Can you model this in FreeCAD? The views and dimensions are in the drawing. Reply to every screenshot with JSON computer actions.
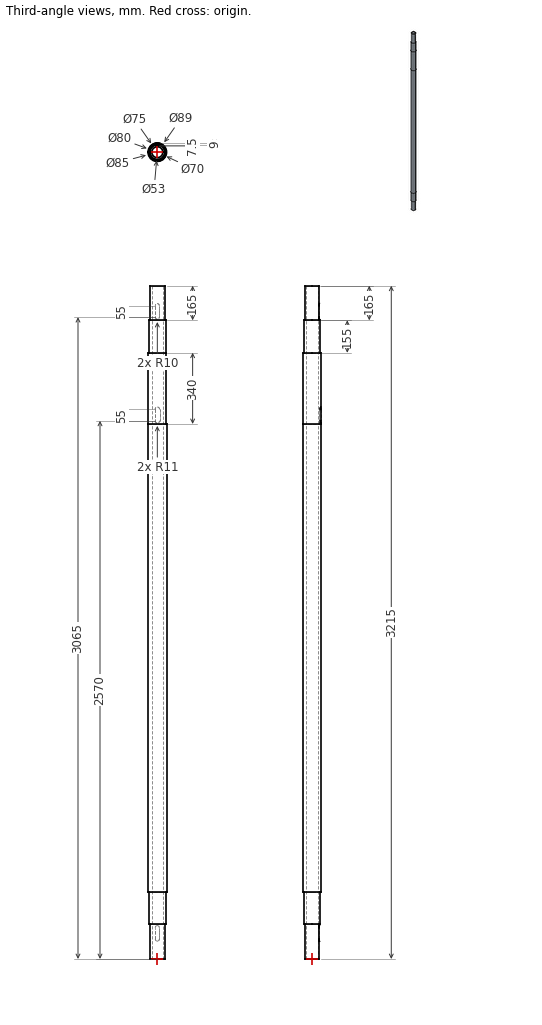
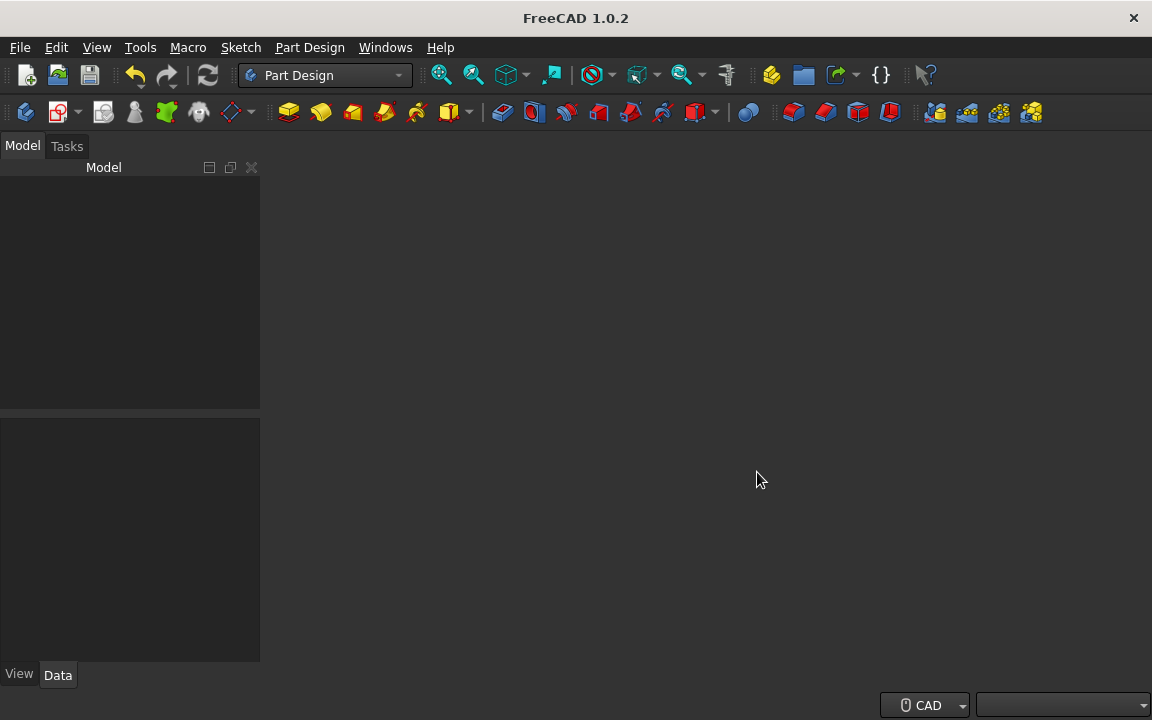
{"action": "left_click", "coordinate": [26, 76]}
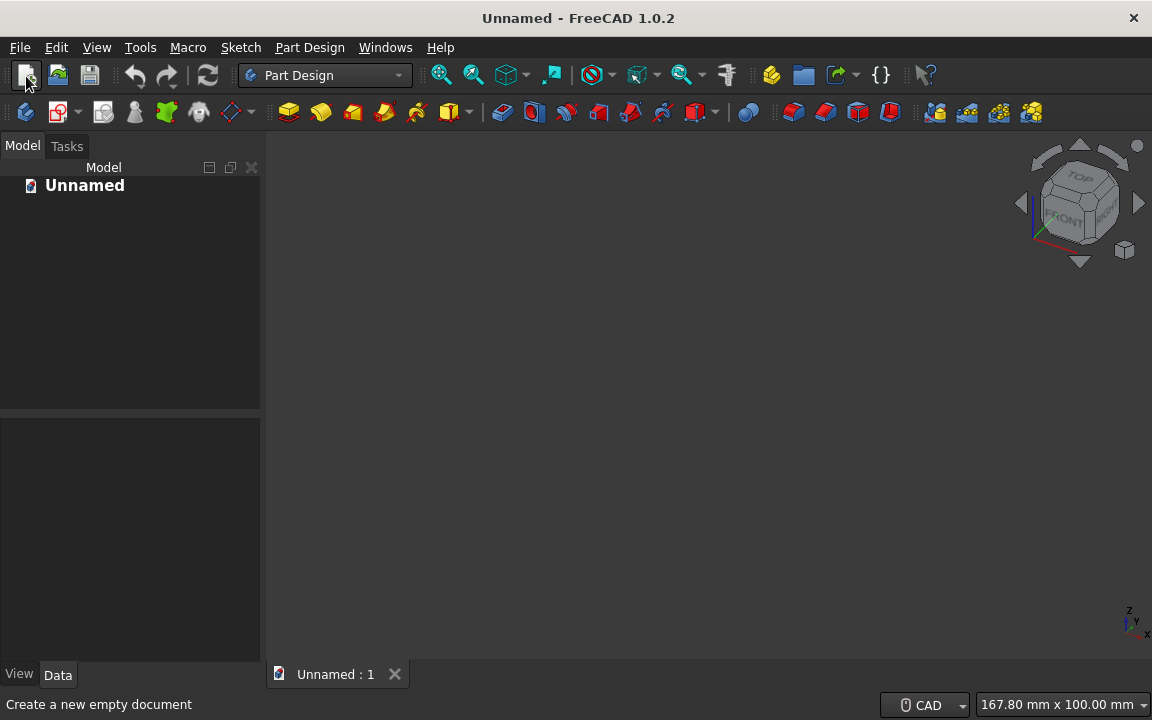
{"action": "left_click", "coordinate": [58, 112]}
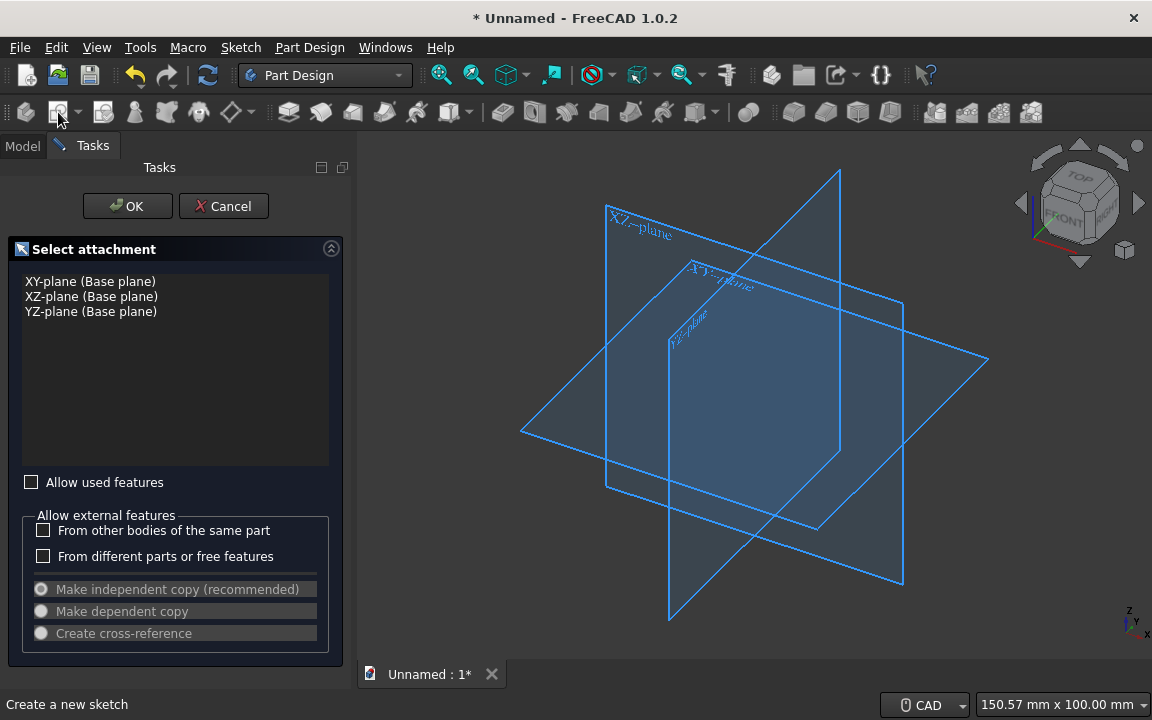
{"action": "left_click", "coordinate": [82, 282]}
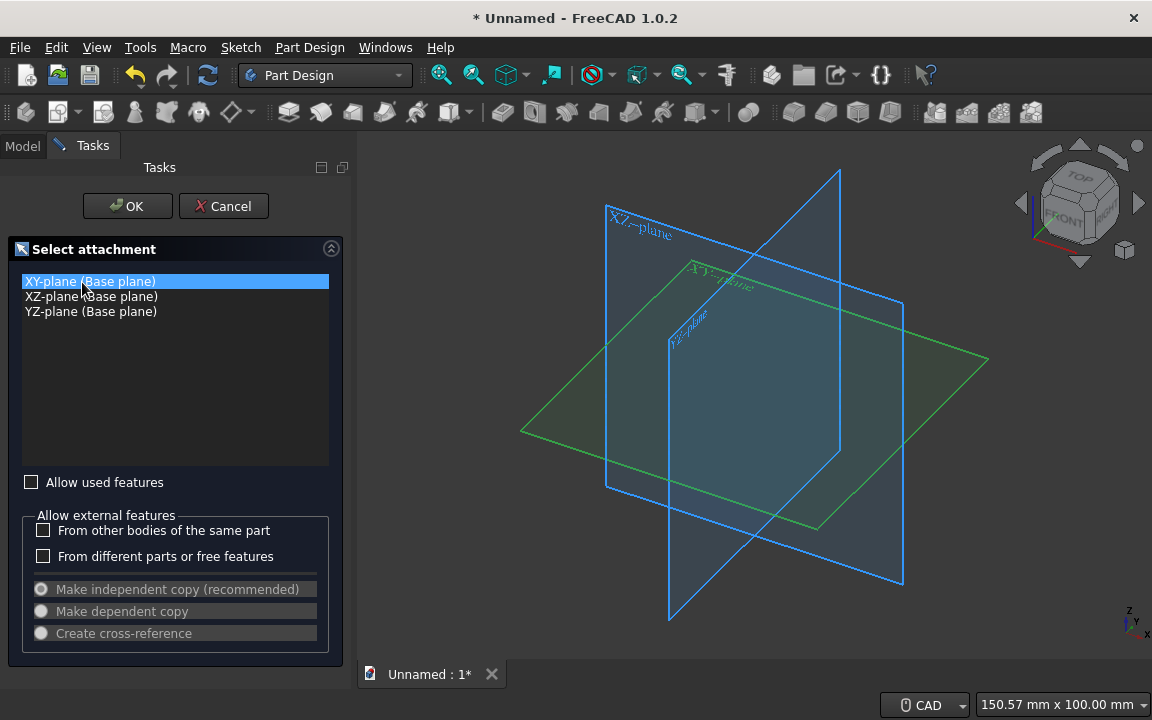
{"action": "left_click", "coordinate": [128, 206]}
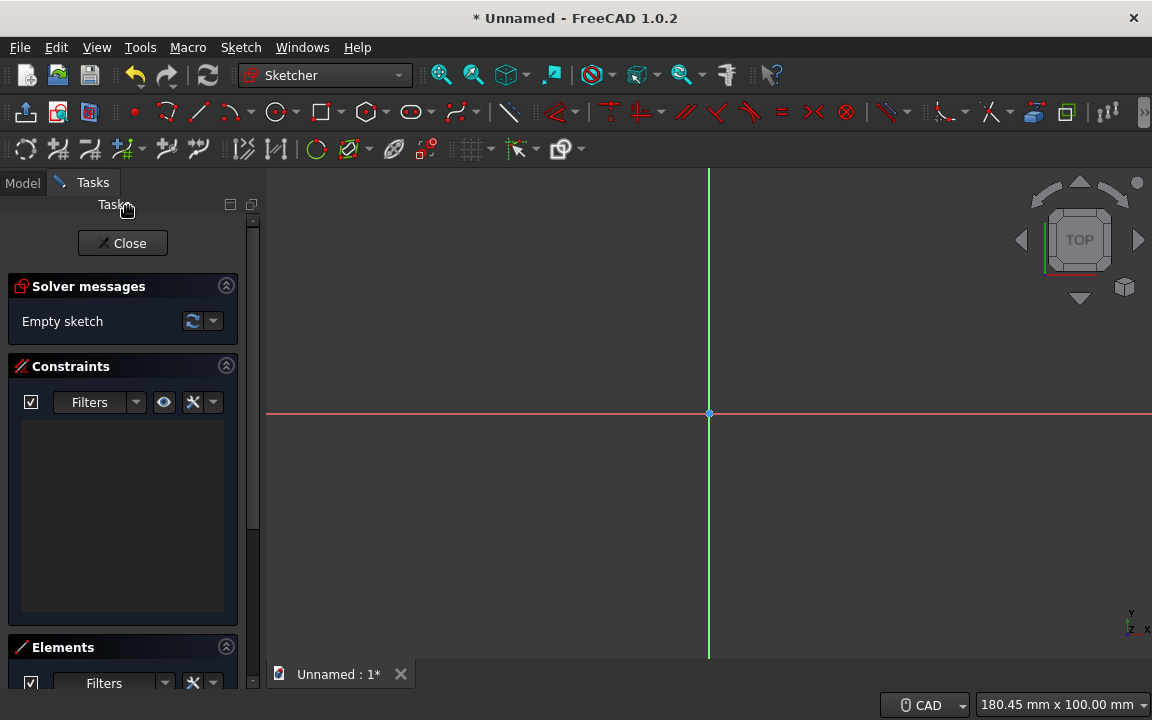
{"action": "scroll", "coordinate": [501, 414], "scroll_direction": "down", "scroll_amount": 2}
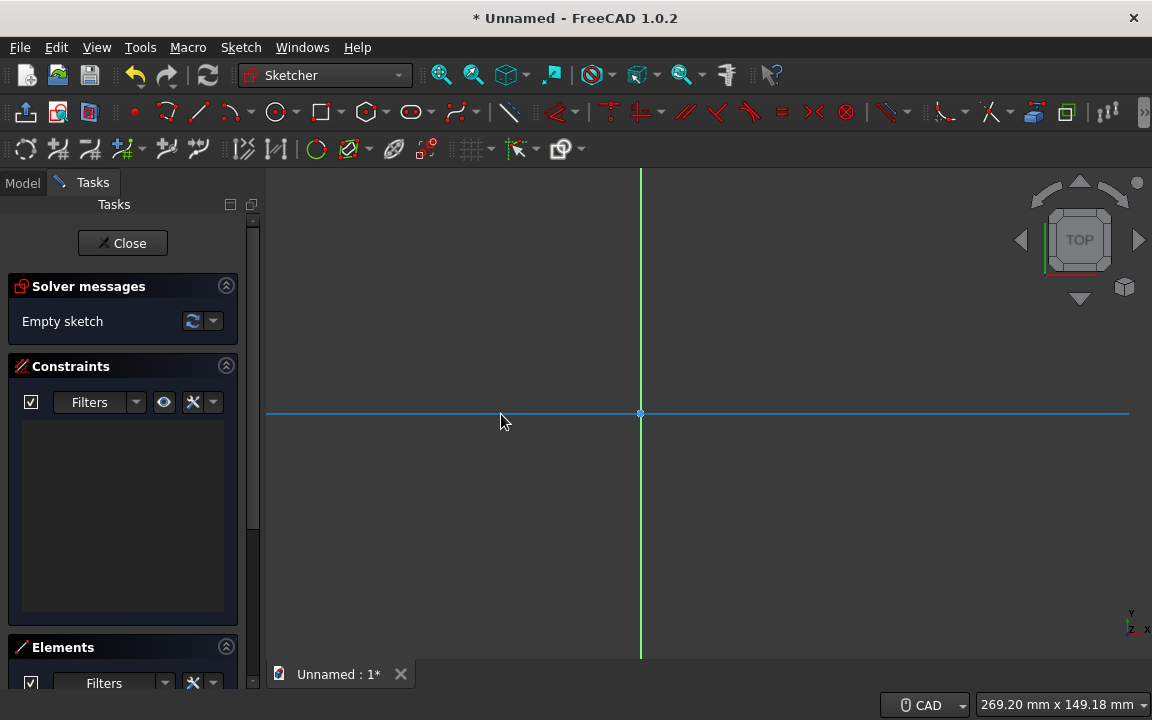
{"action": "left_click", "coordinate": [276, 112]}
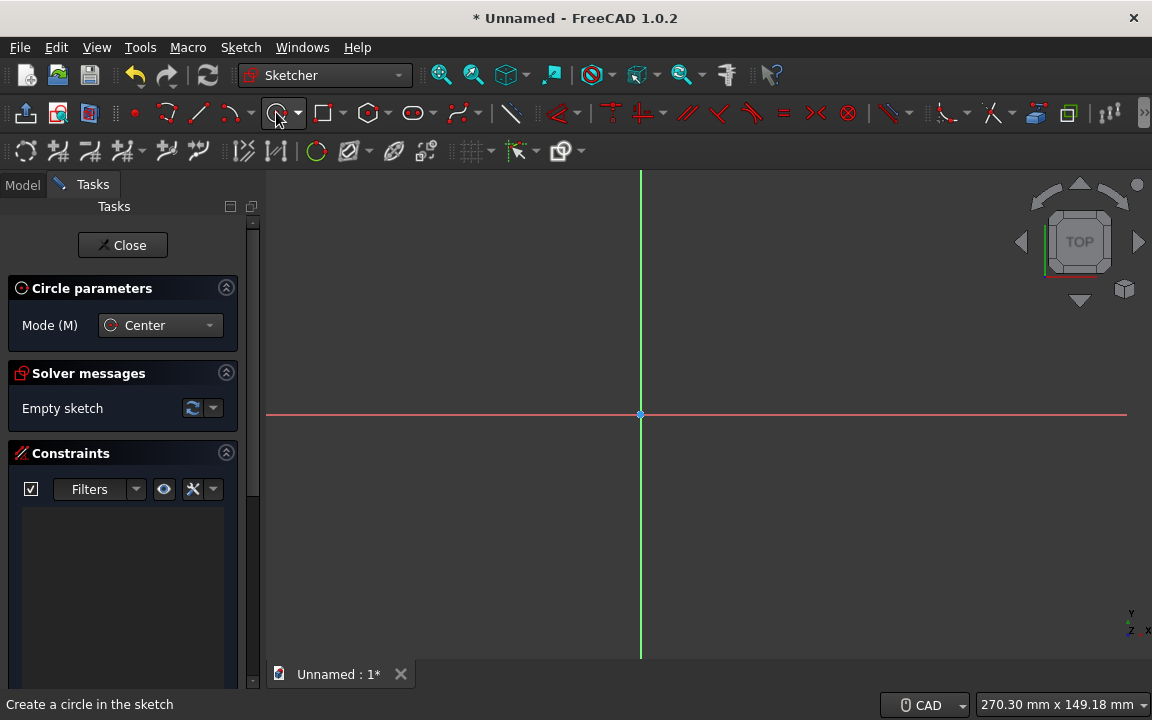
{"action": "left_click", "coordinate": [641, 415]}
{"action": "mouse_move", "coordinate": [744, 312]}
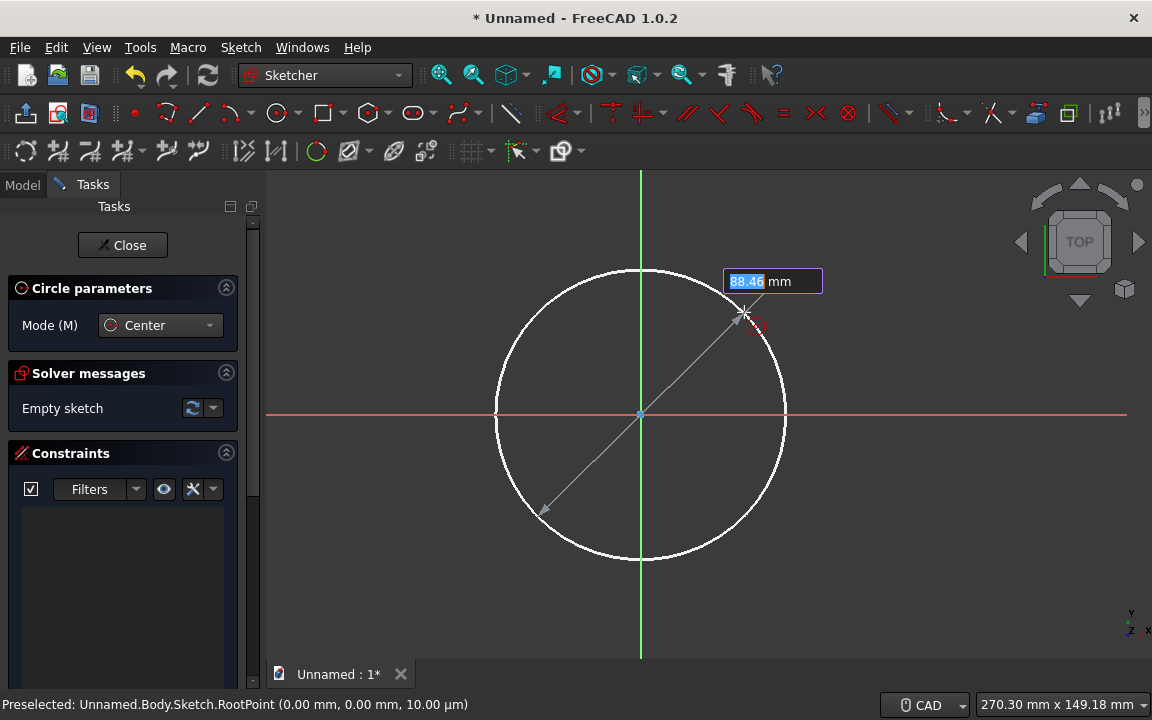
{"action": "type", "text": "89"}
{"action": "key", "text": "Return"}
{"action": "key", "text": "Escape"}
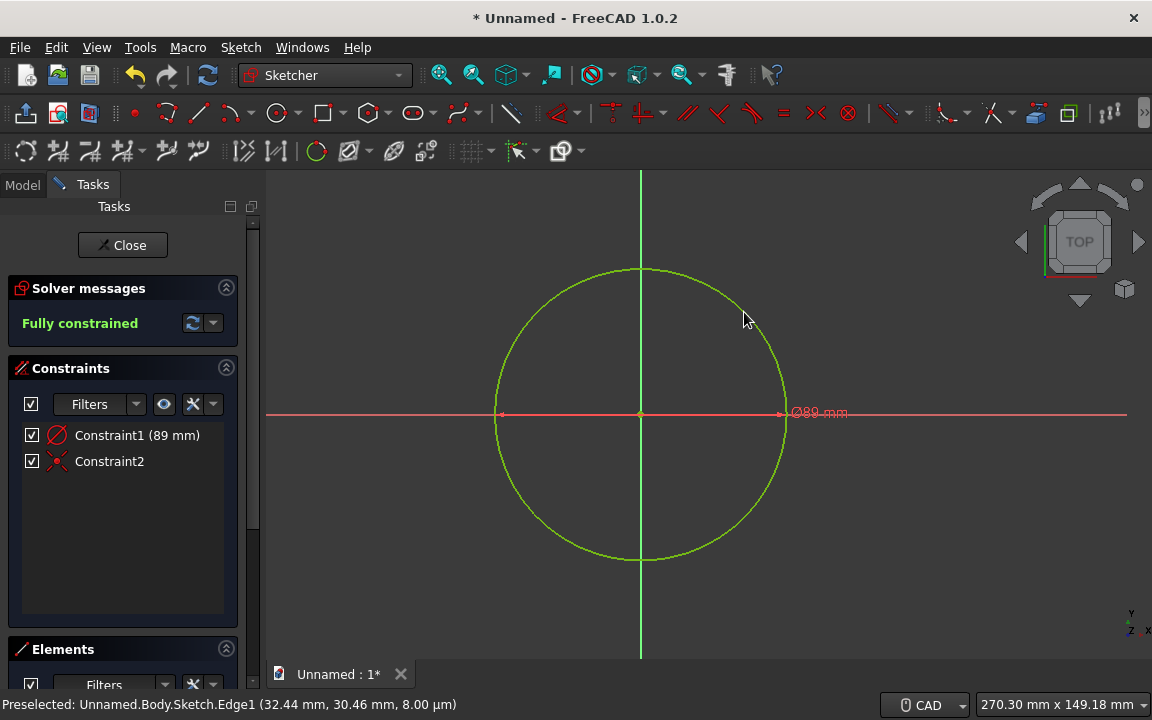
{"action": "left_click", "coordinate": [123, 245]}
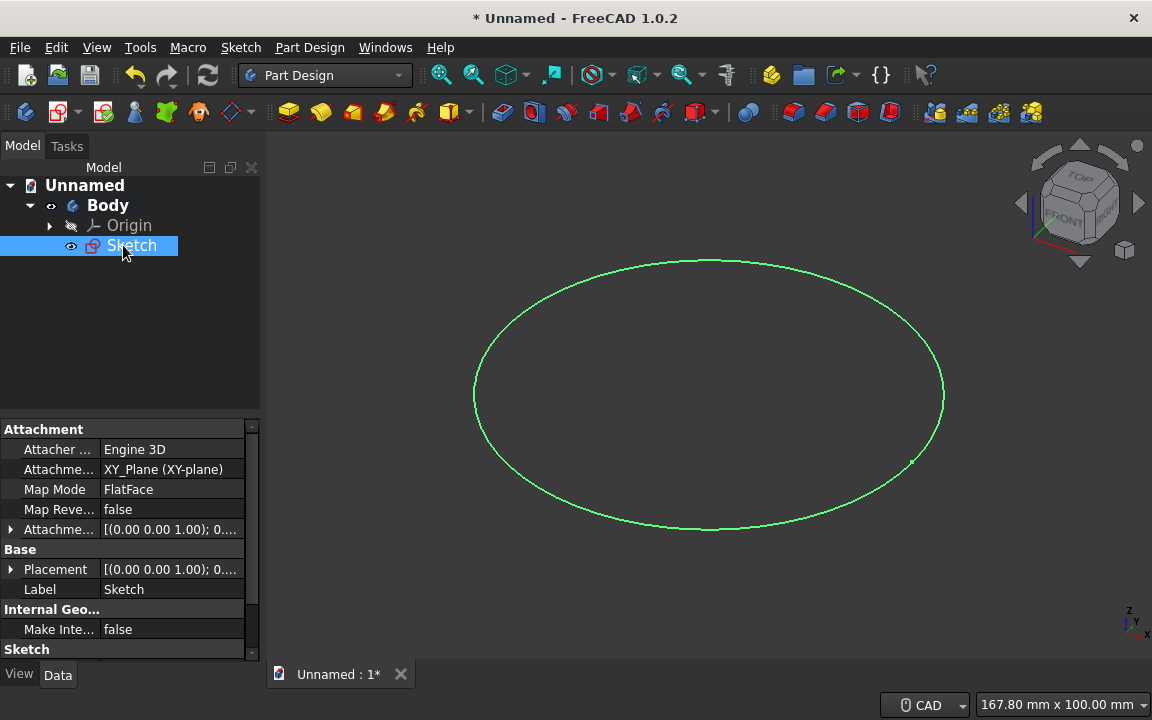
{"action": "left_click", "coordinate": [290, 112]}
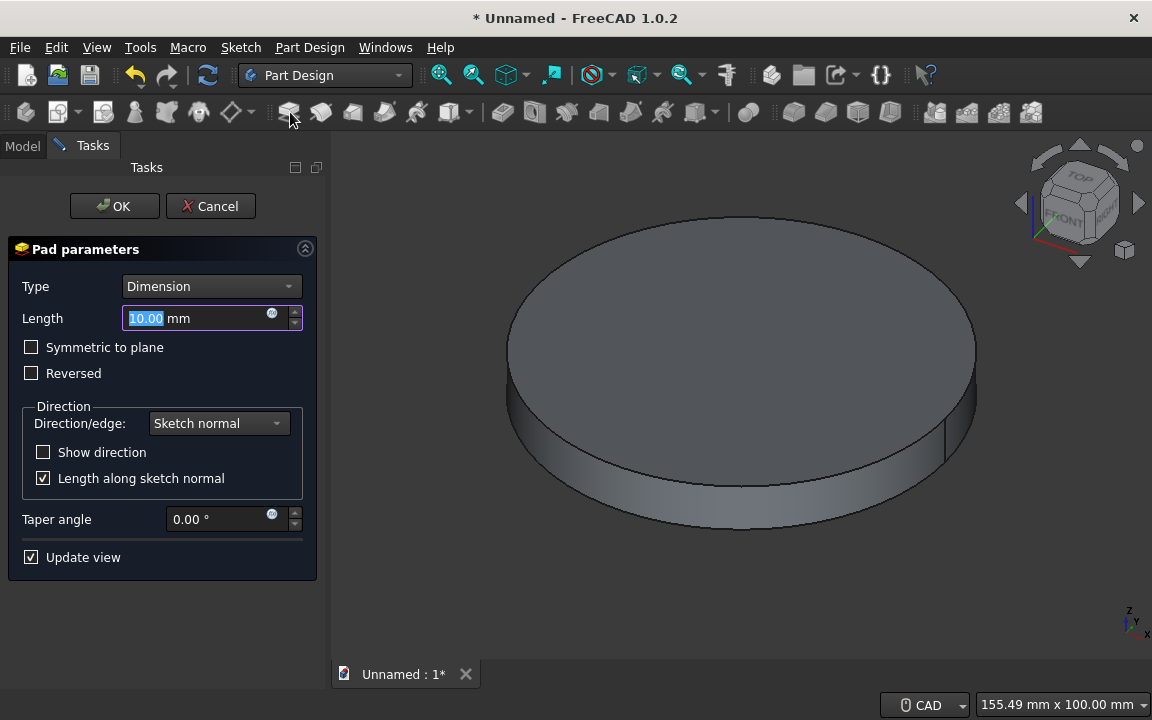
{"action": "type", "text": "3215"}
{"action": "key", "text": "Tab"}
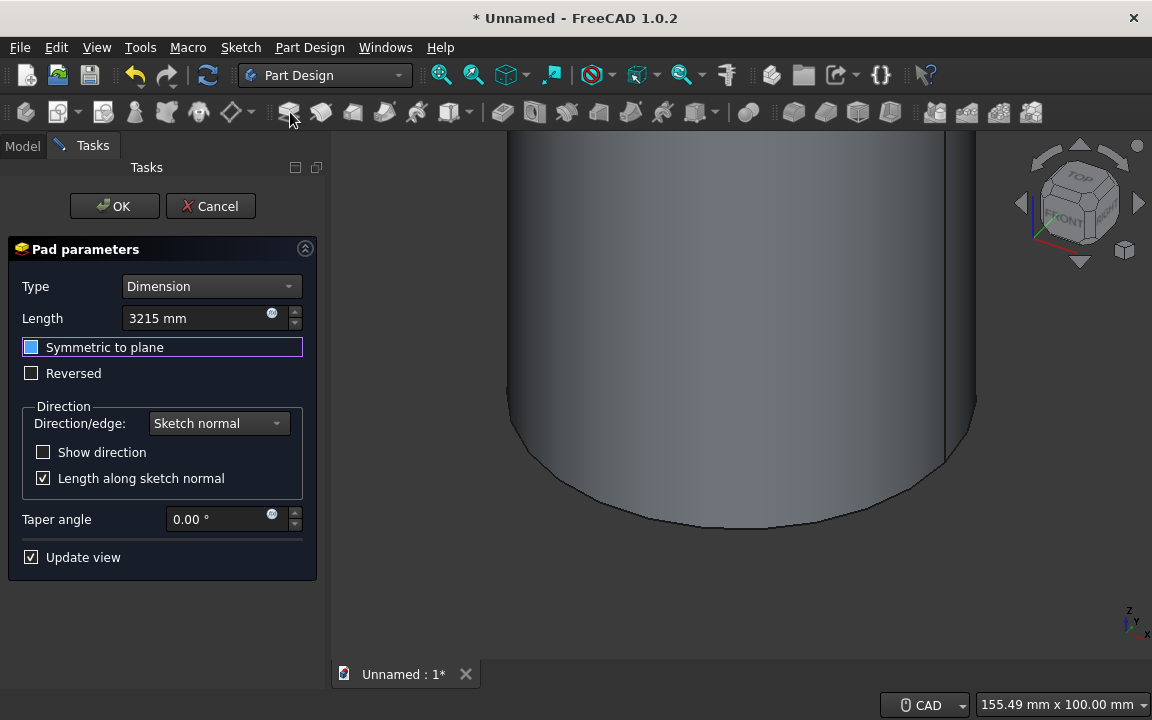
{"action": "left_click", "coordinate": [115, 206]}